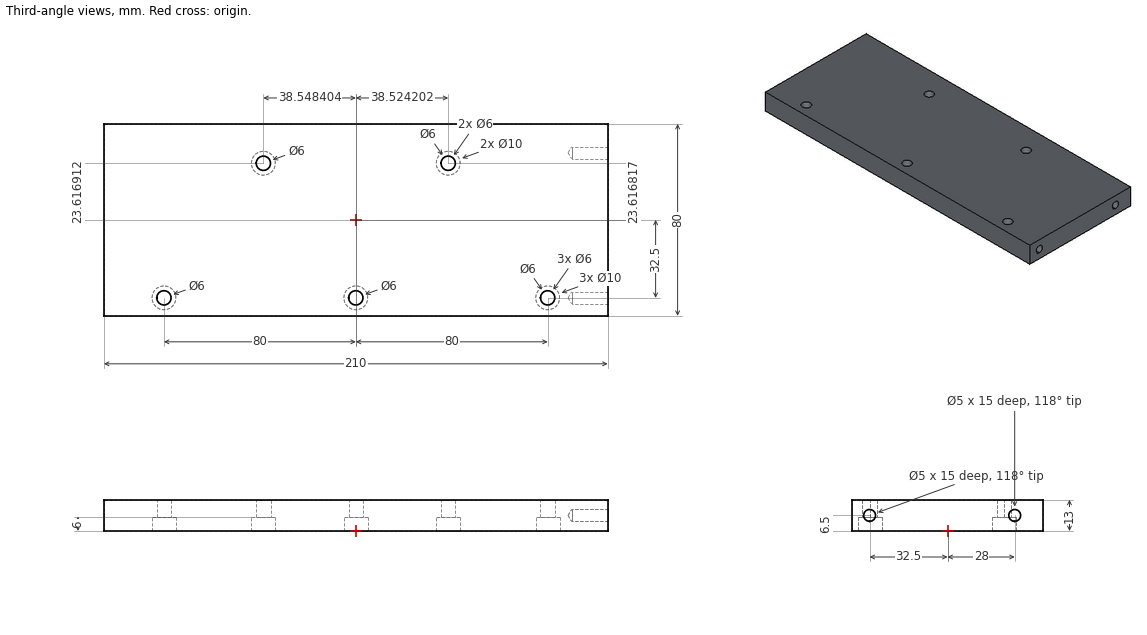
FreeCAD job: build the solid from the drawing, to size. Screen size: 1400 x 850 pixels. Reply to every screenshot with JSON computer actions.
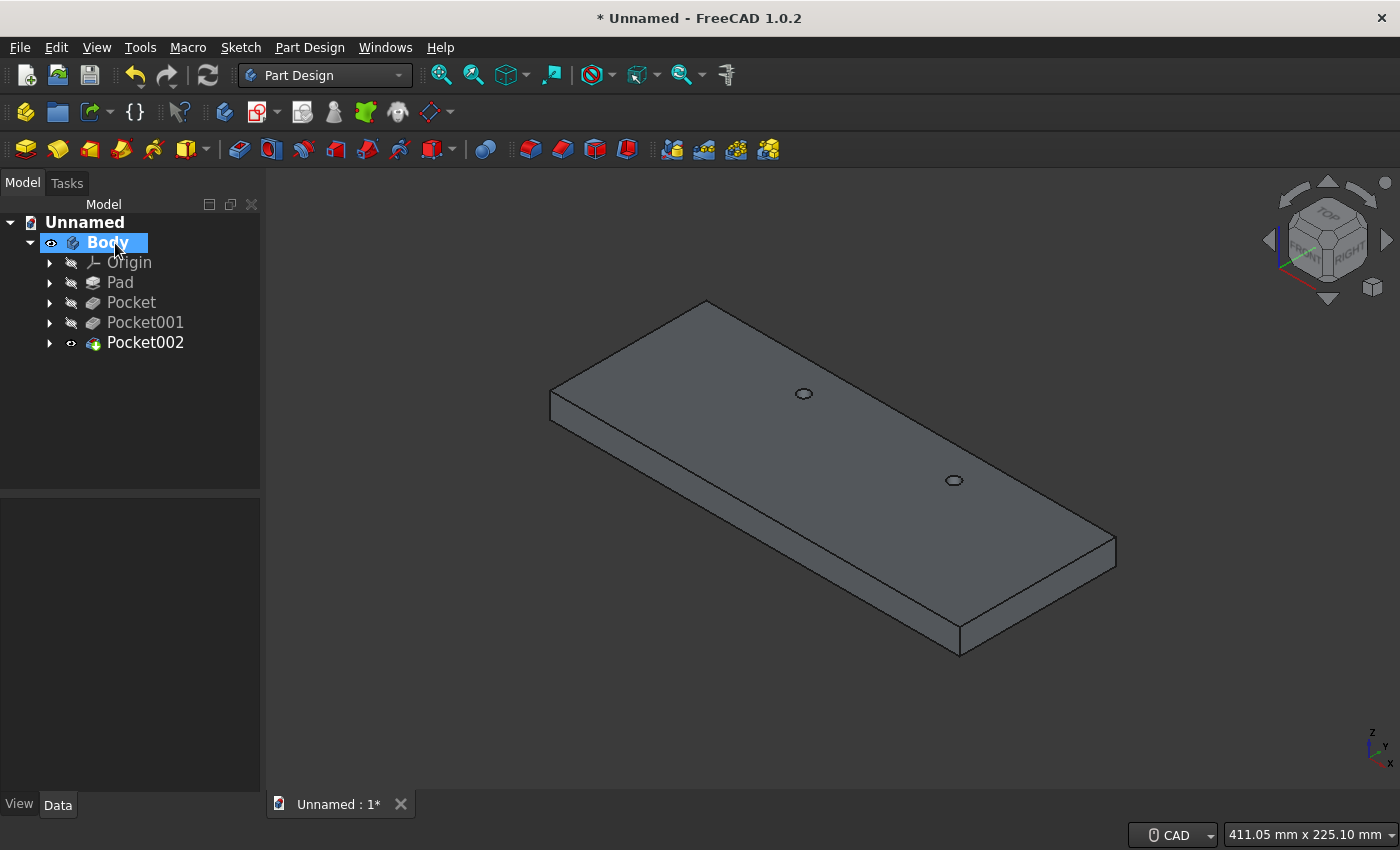
{"action": "left_click", "coordinate": [1082, 570]}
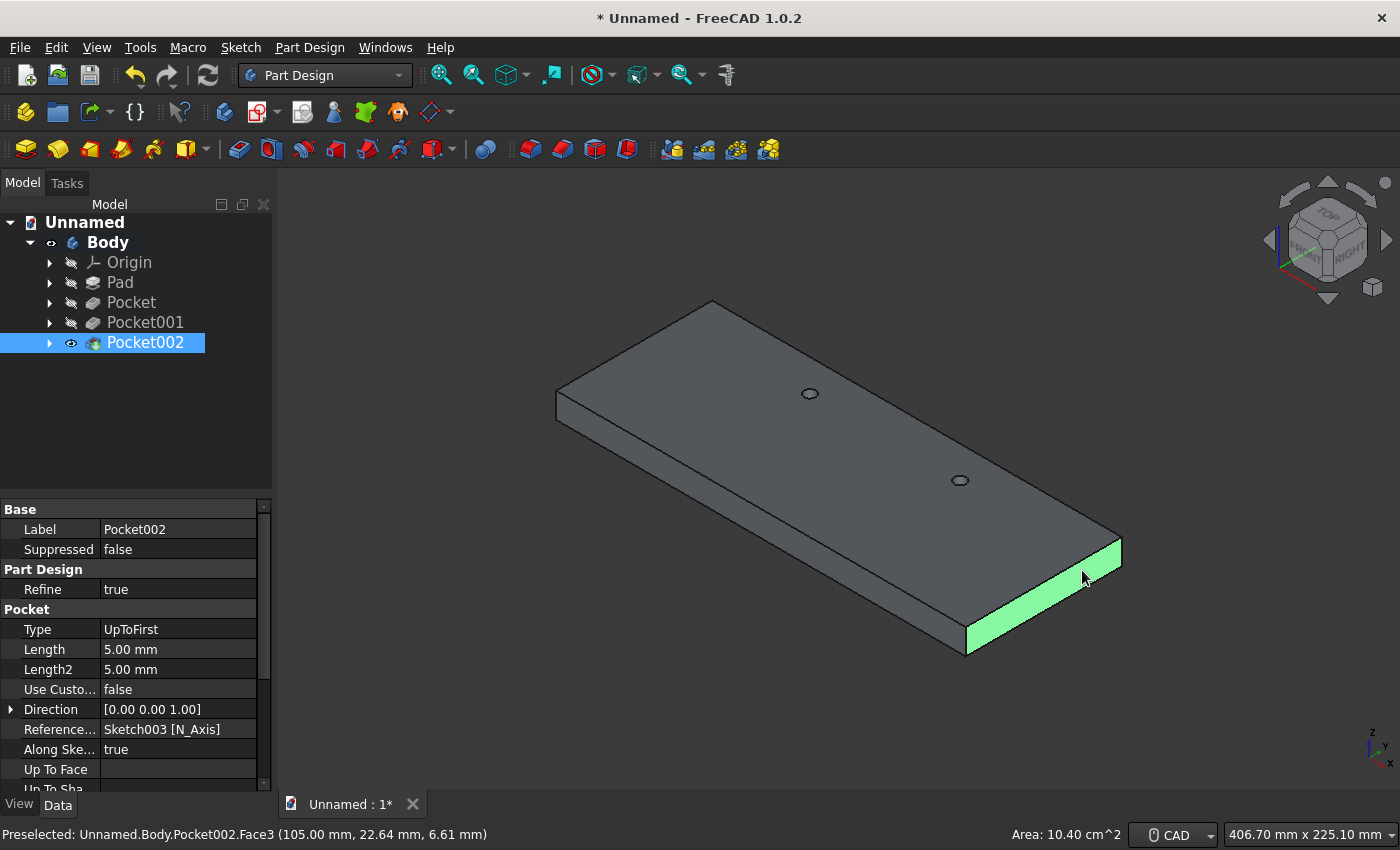
{"action": "left_click", "coordinate": [258, 112]}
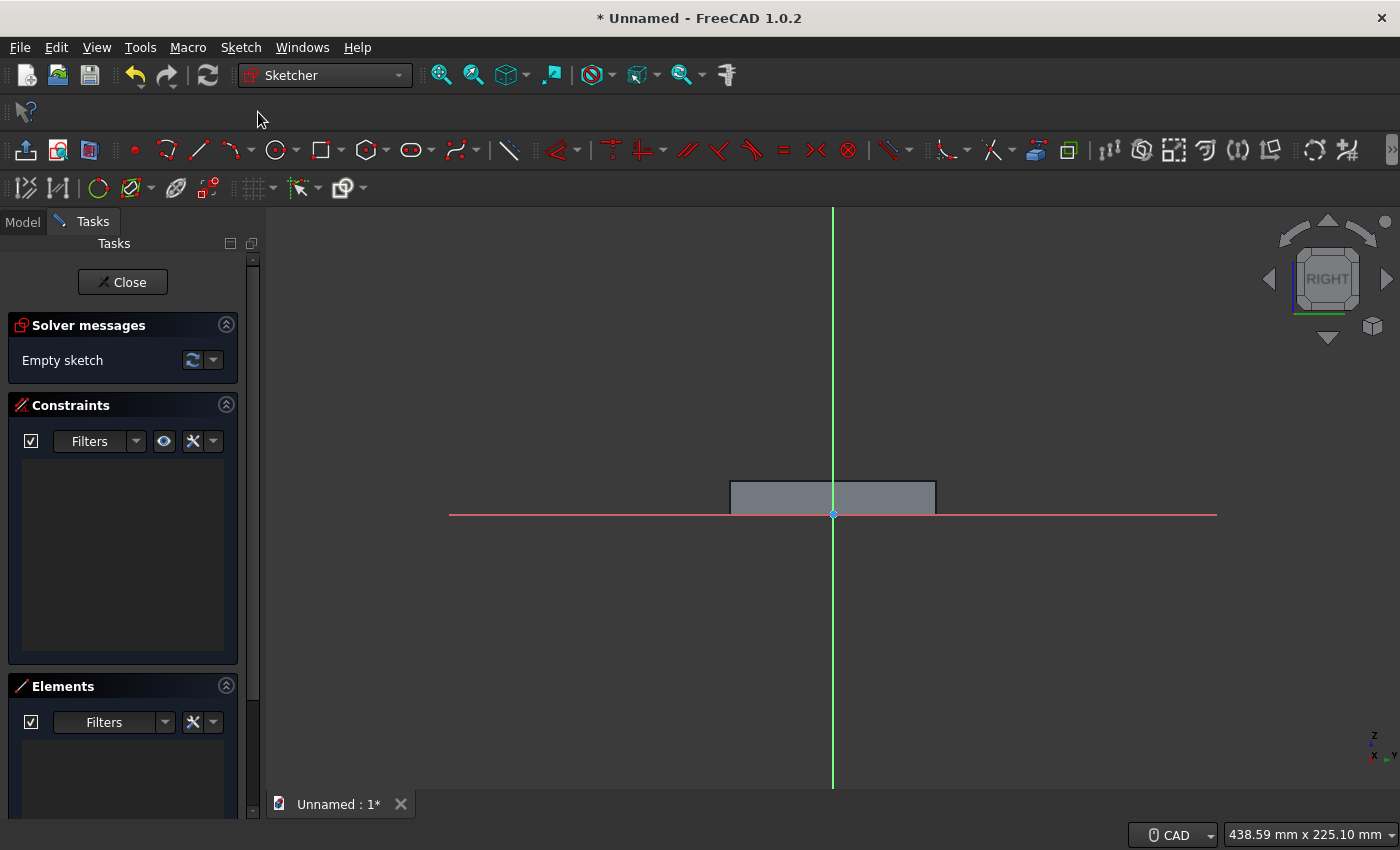
{"action": "scroll", "coordinate": [748, 498], "scroll_direction": "up", "scroll_amount": 15}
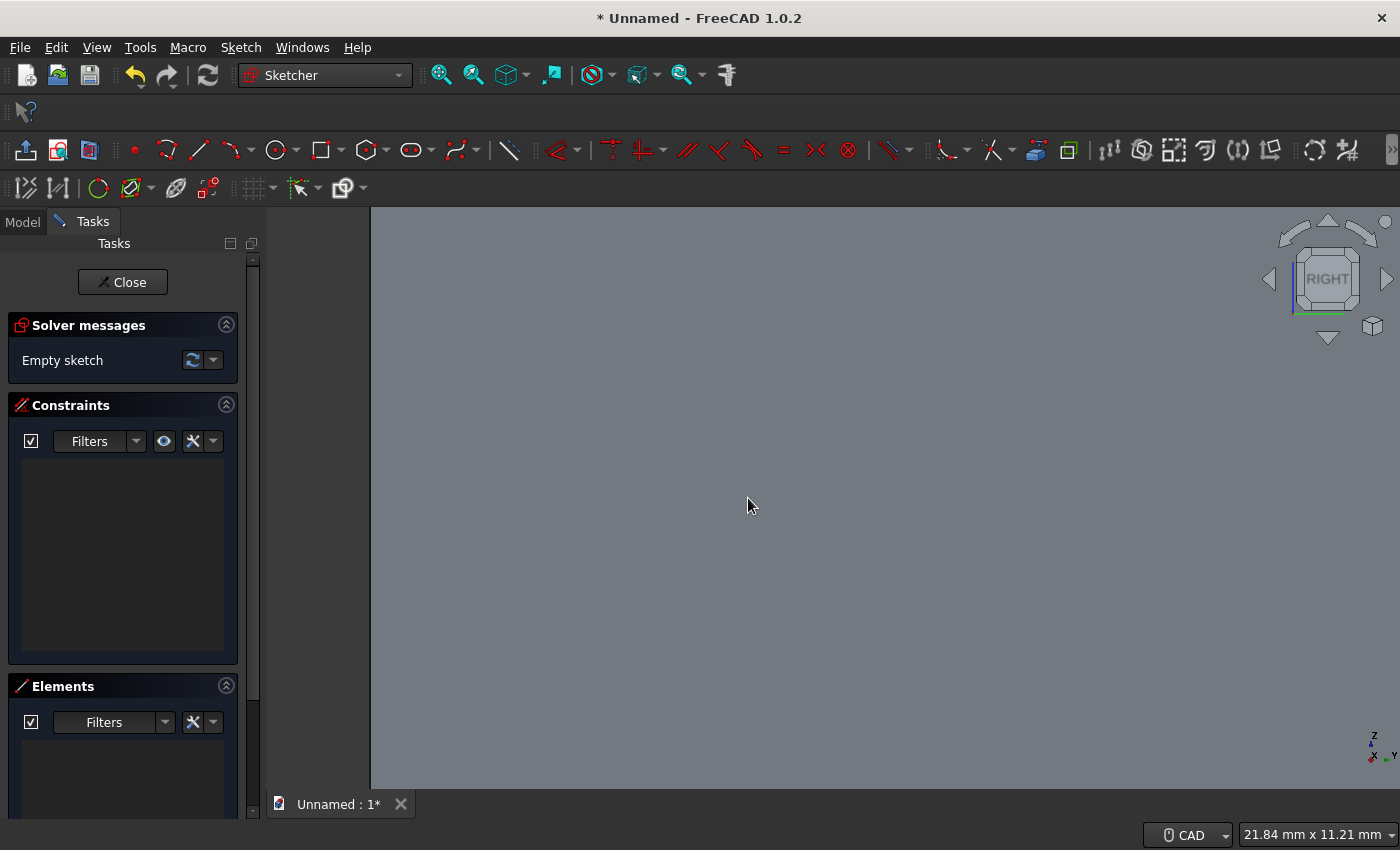
{"action": "scroll", "coordinate": [749, 469], "scroll_direction": "up", "scroll_amount": 2}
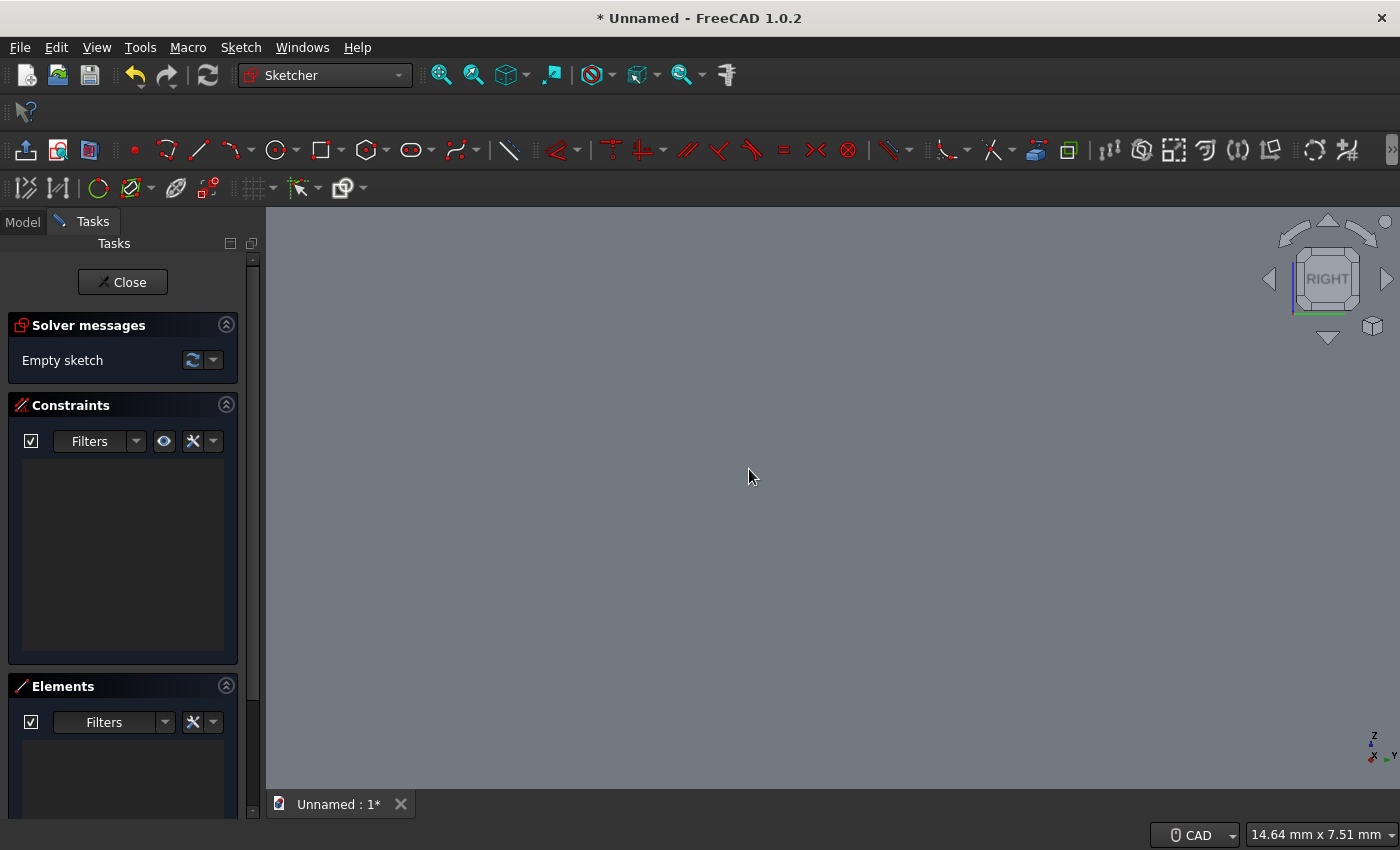
{"action": "key", "text": "g c"}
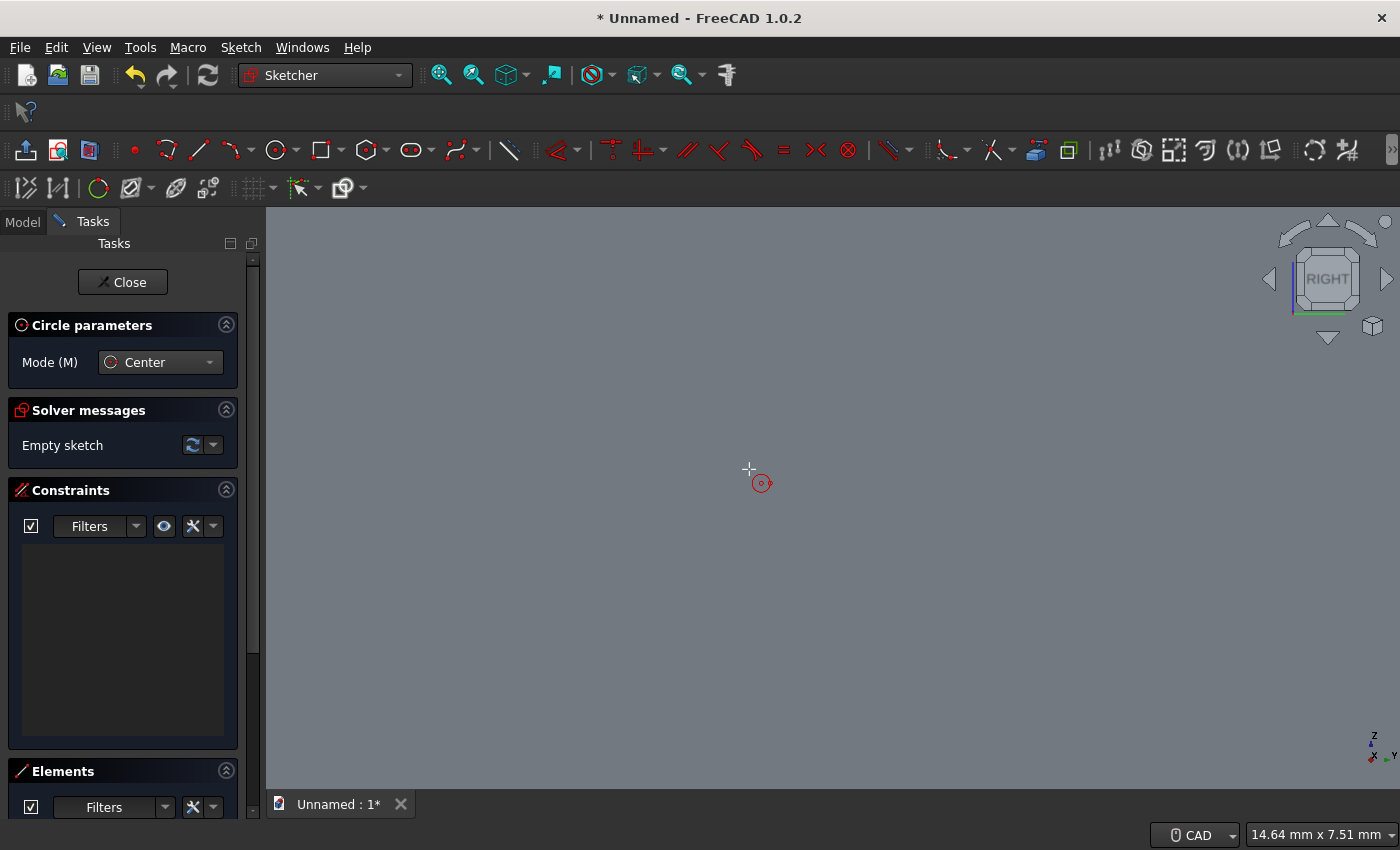
{"action": "left_click", "coordinate": [764, 498]}
{"action": "left_click", "coordinate": [901, 361]}
{"action": "key", "text": "Escape"}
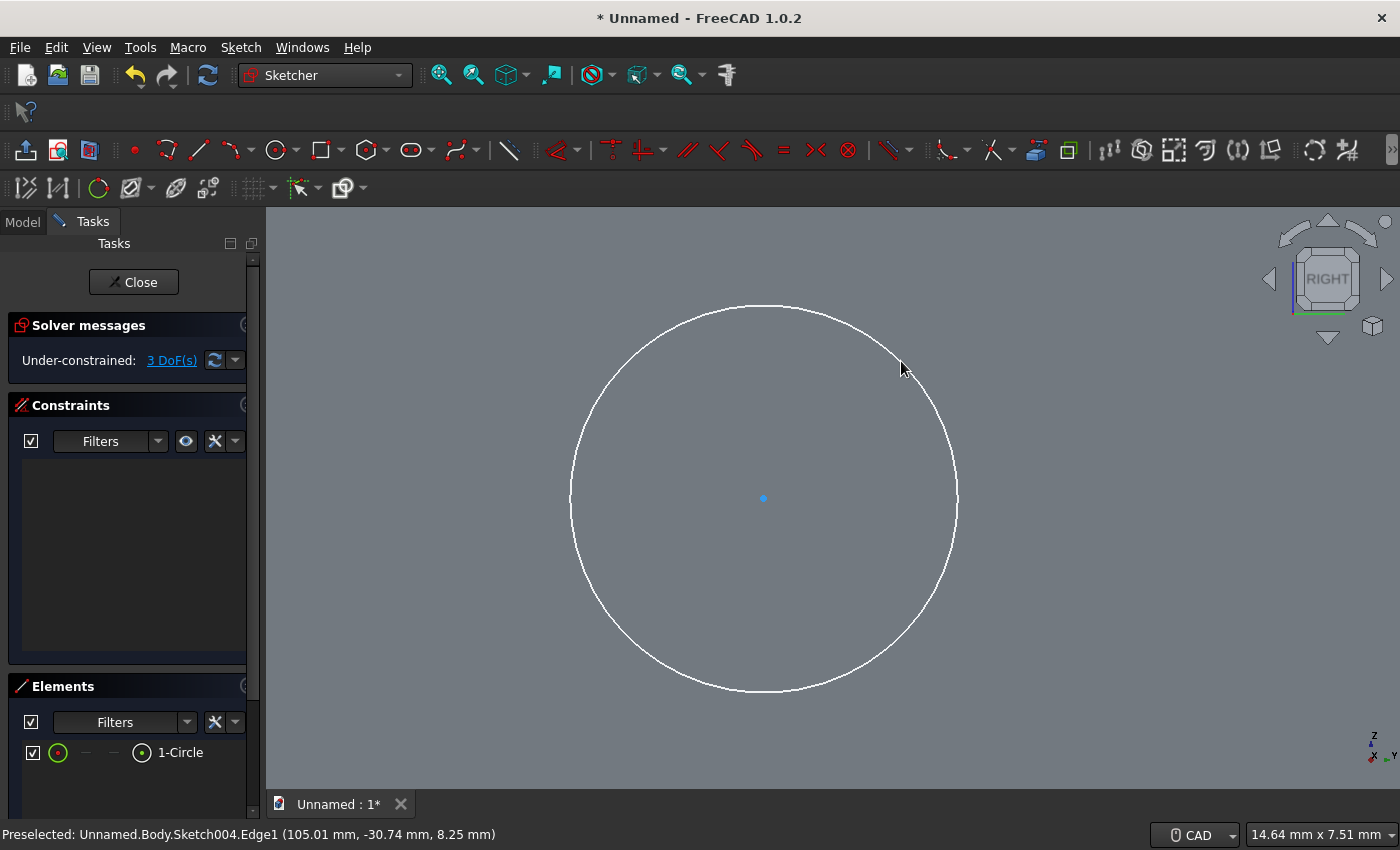
{"action": "key", "text": "d"}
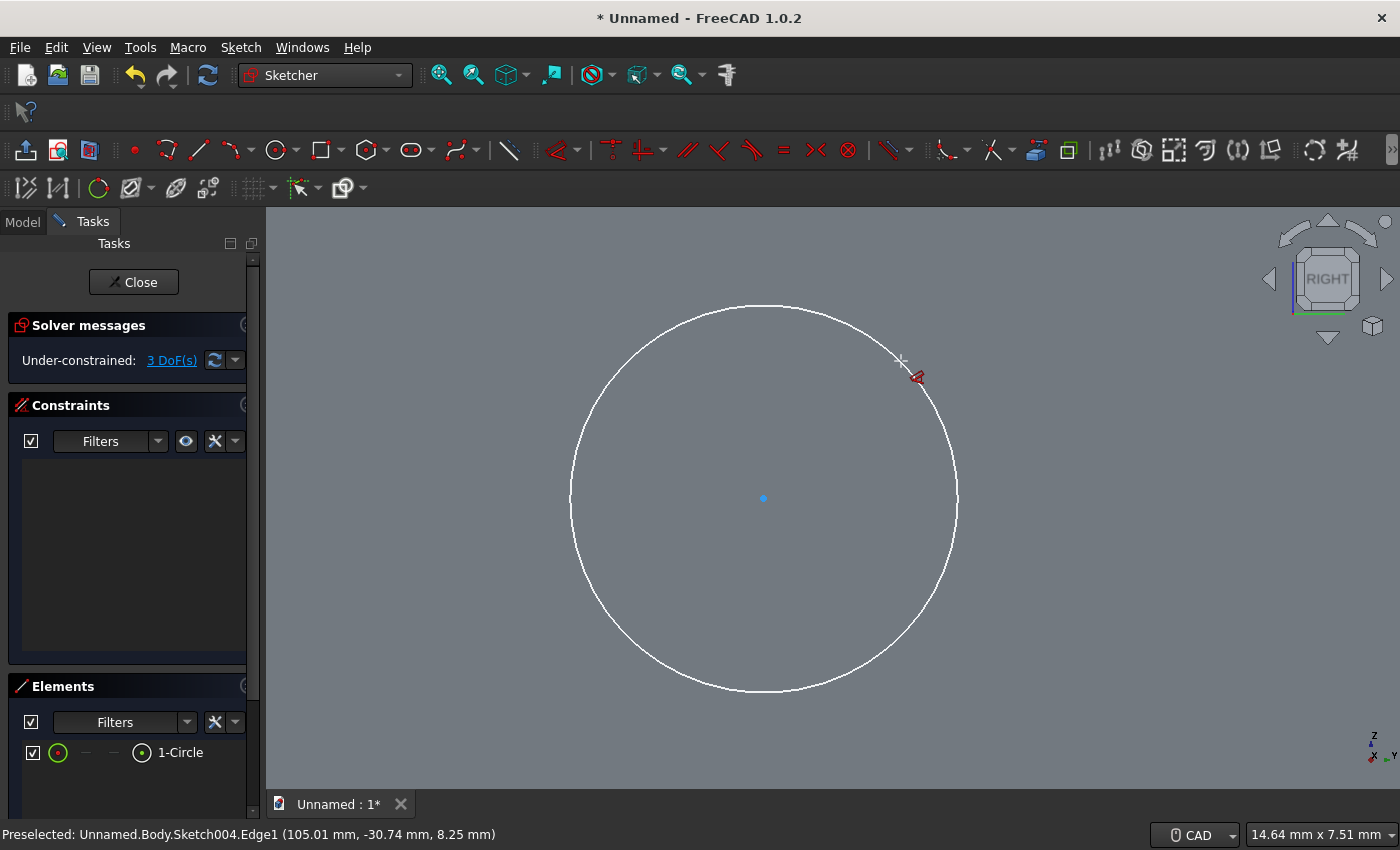
{"action": "left_click", "coordinate": [901, 362]}
{"action": "left_click", "coordinate": [924, 339]}